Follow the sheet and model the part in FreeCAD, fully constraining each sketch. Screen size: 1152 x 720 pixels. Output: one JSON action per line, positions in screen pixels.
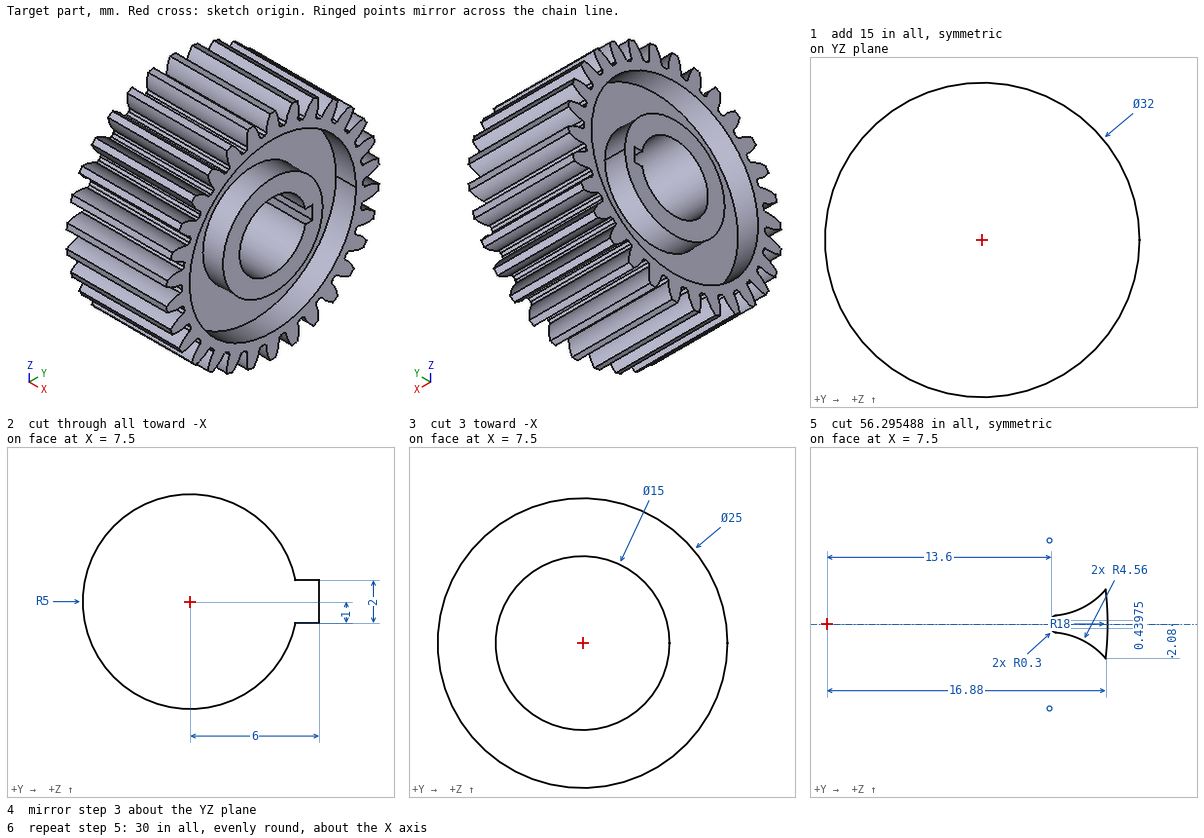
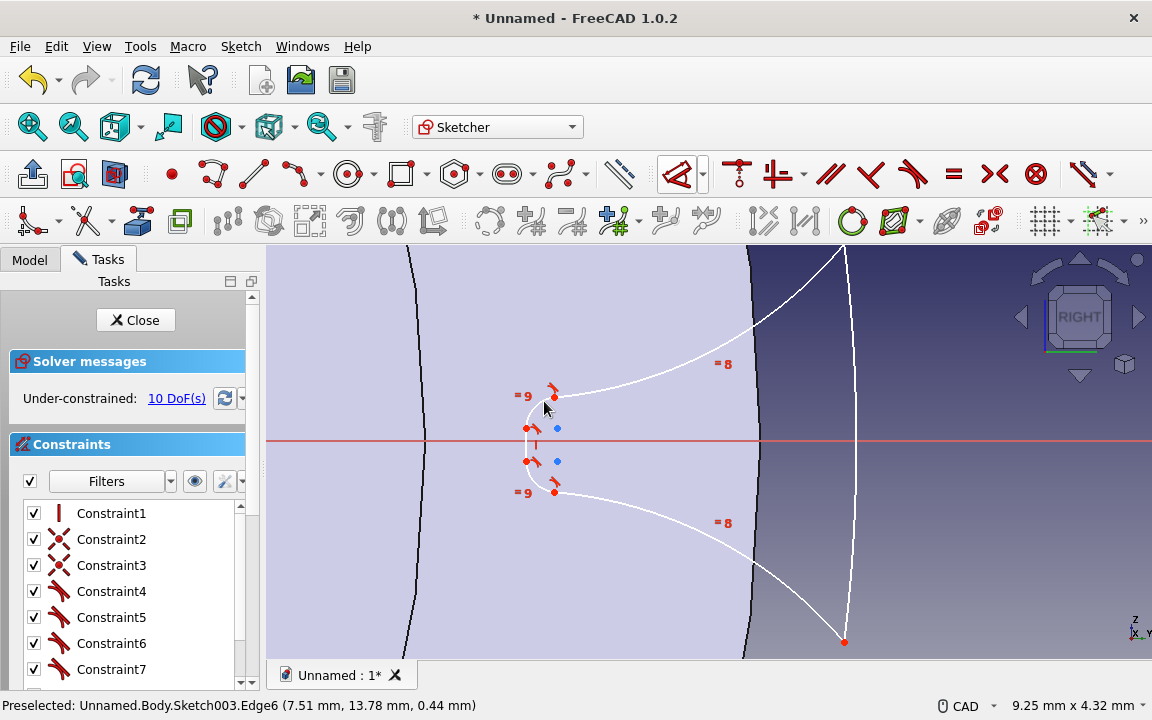
{"action": "scroll", "coordinate": [533, 474], "scroll_direction": "down", "scroll_amount": 2}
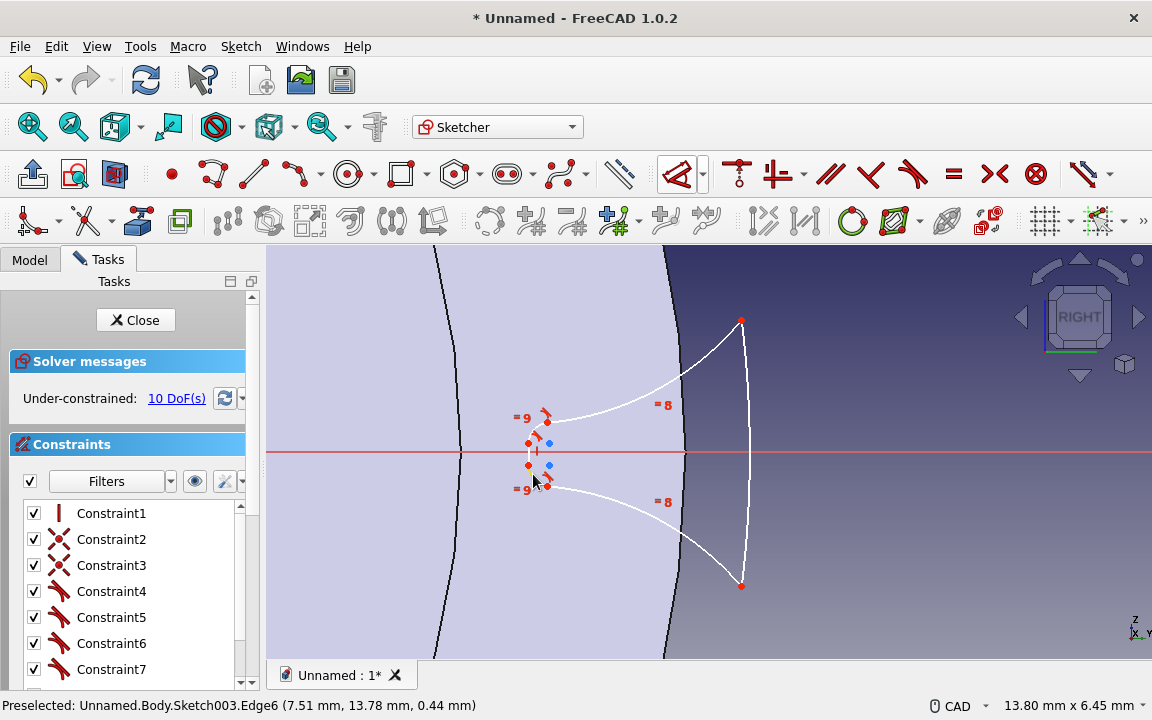
{"action": "scroll", "coordinate": [987, 452], "scroll_direction": "down", "scroll_amount": 4}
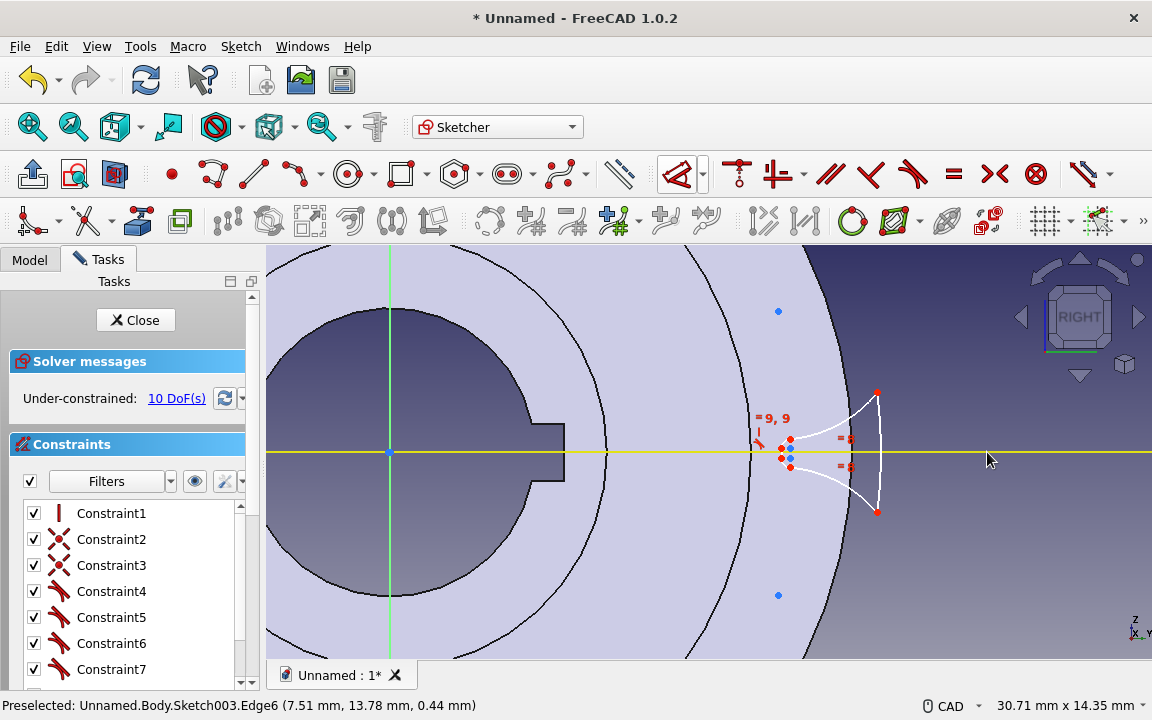
{"action": "scroll", "coordinate": [388, 453], "scroll_direction": "up", "scroll_amount": 9}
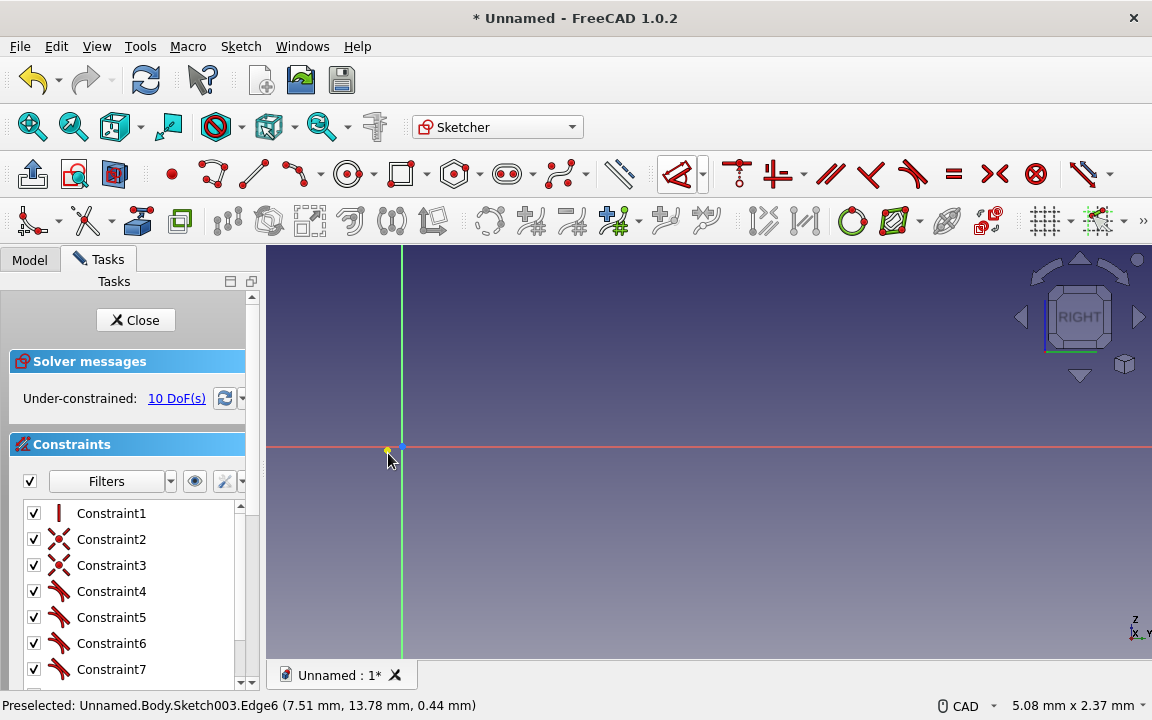
{"action": "left_click", "coordinate": [388, 450]}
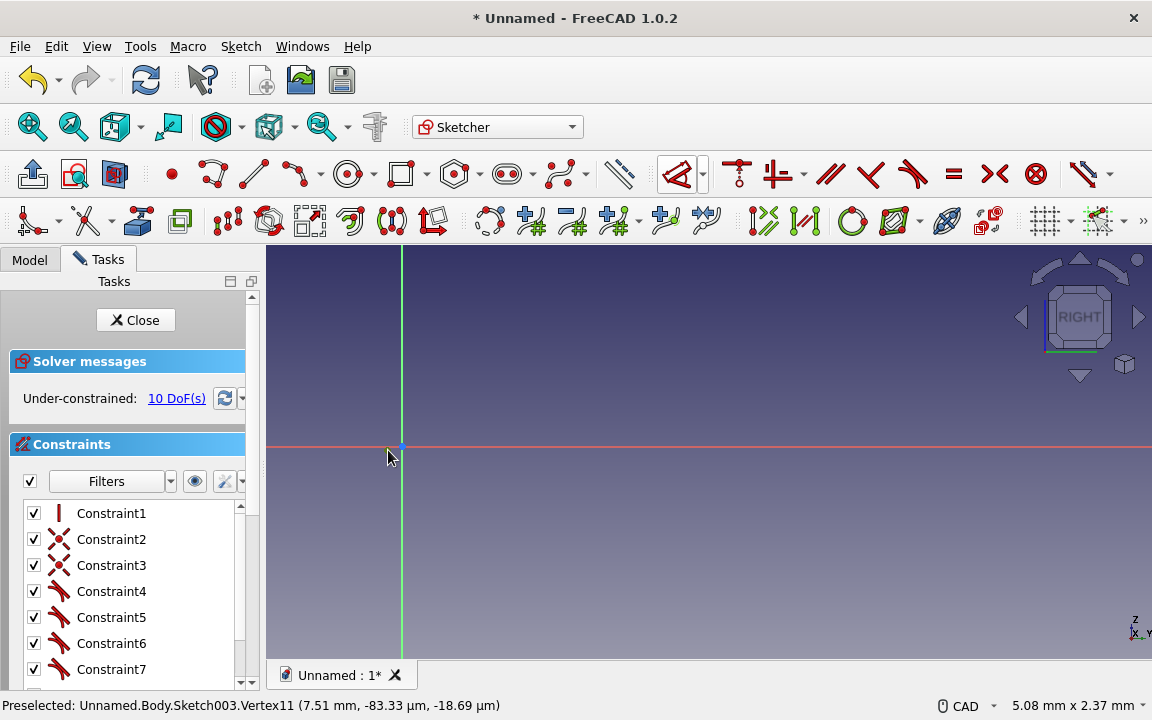
{"action": "left_click", "coordinate": [344, 447]}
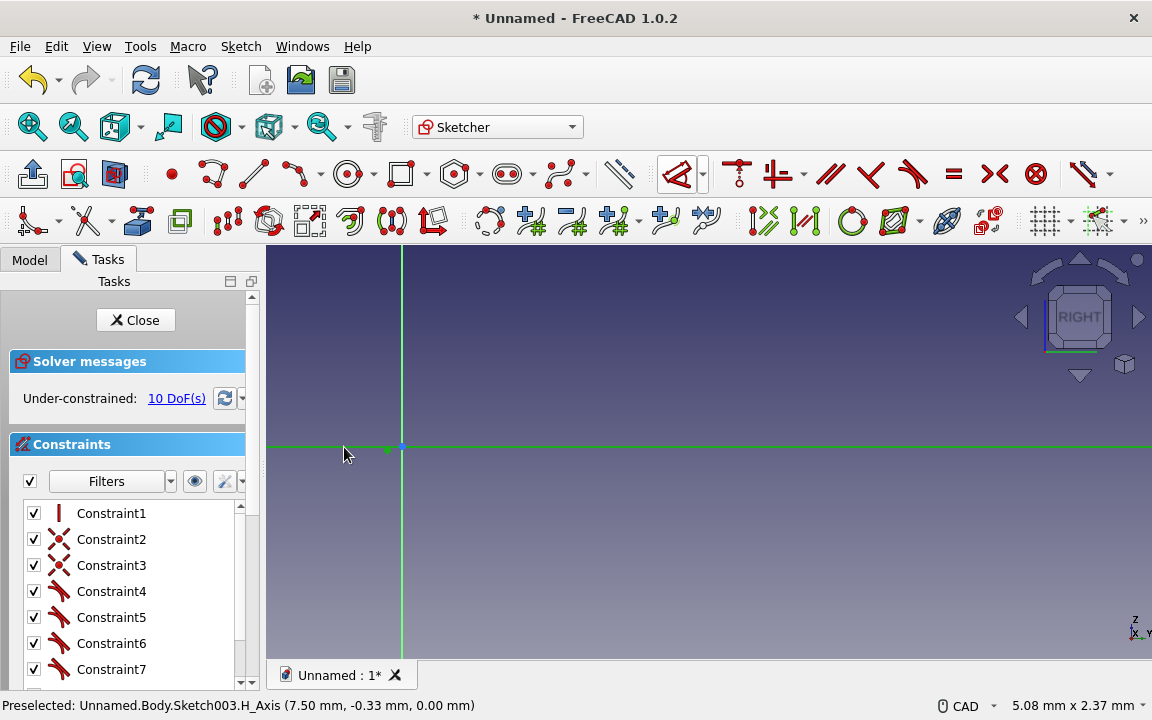
{"action": "key", "text": "c"}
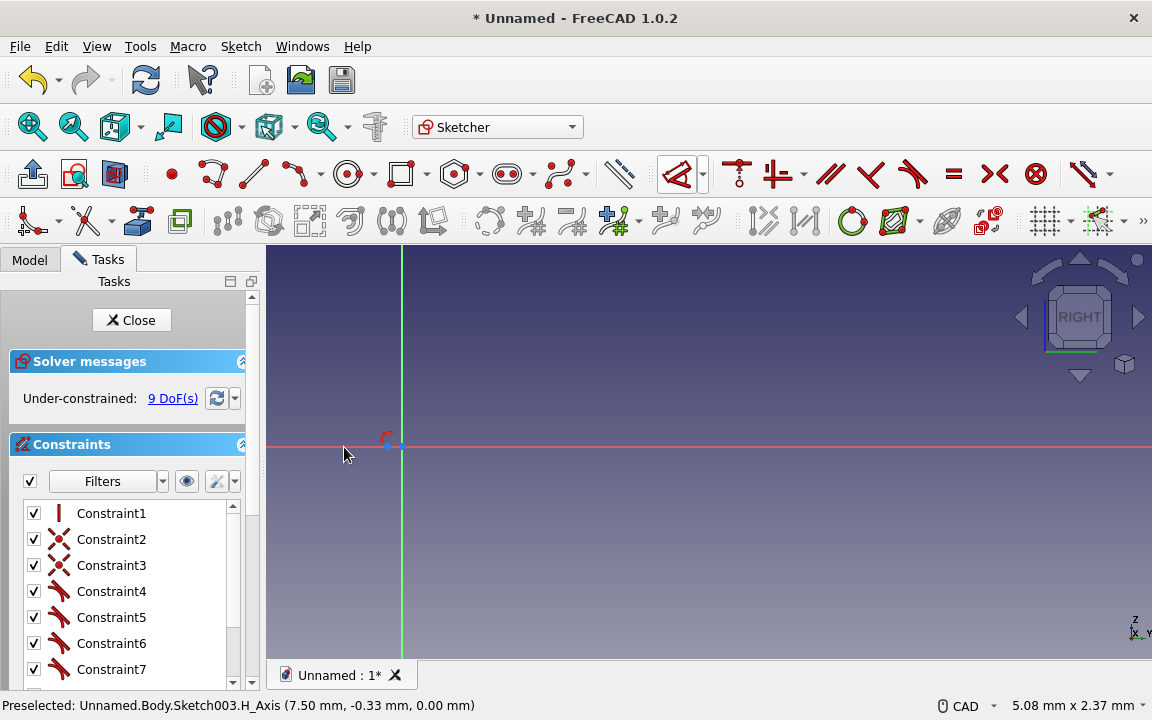
{"action": "scroll", "coordinate": [294, 453], "scroll_direction": "down", "scroll_amount": 8}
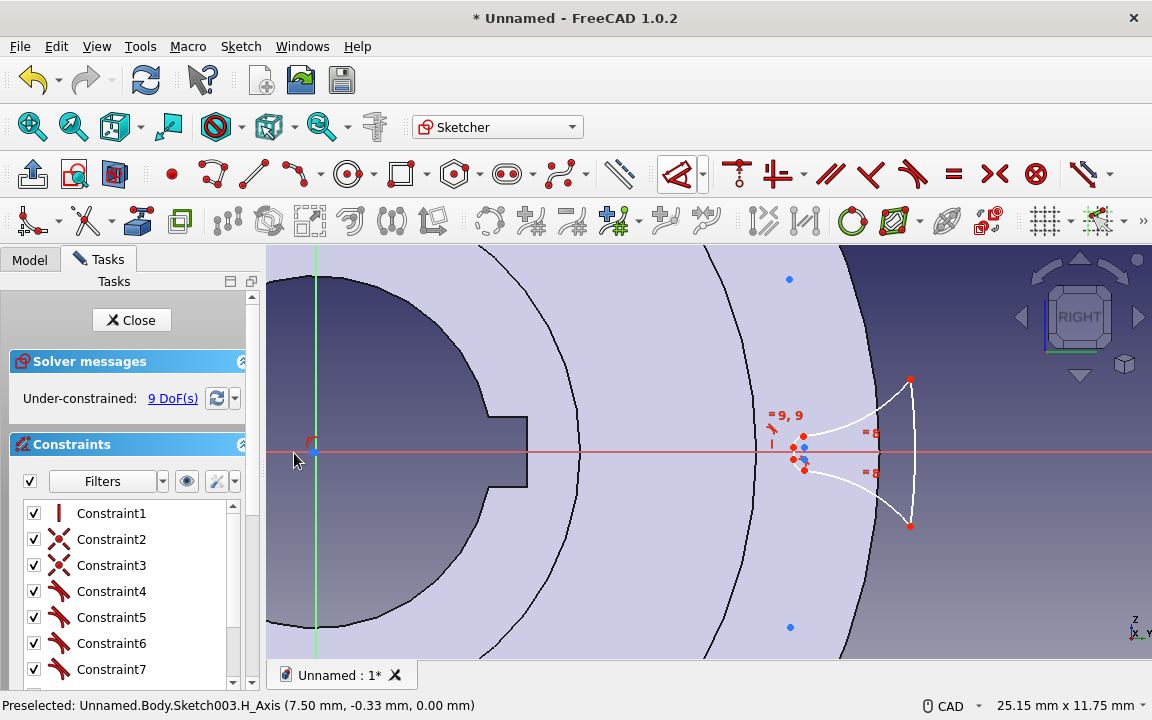
{"action": "scroll", "coordinate": [987, 452], "scroll_direction": "up", "scroll_amount": 3}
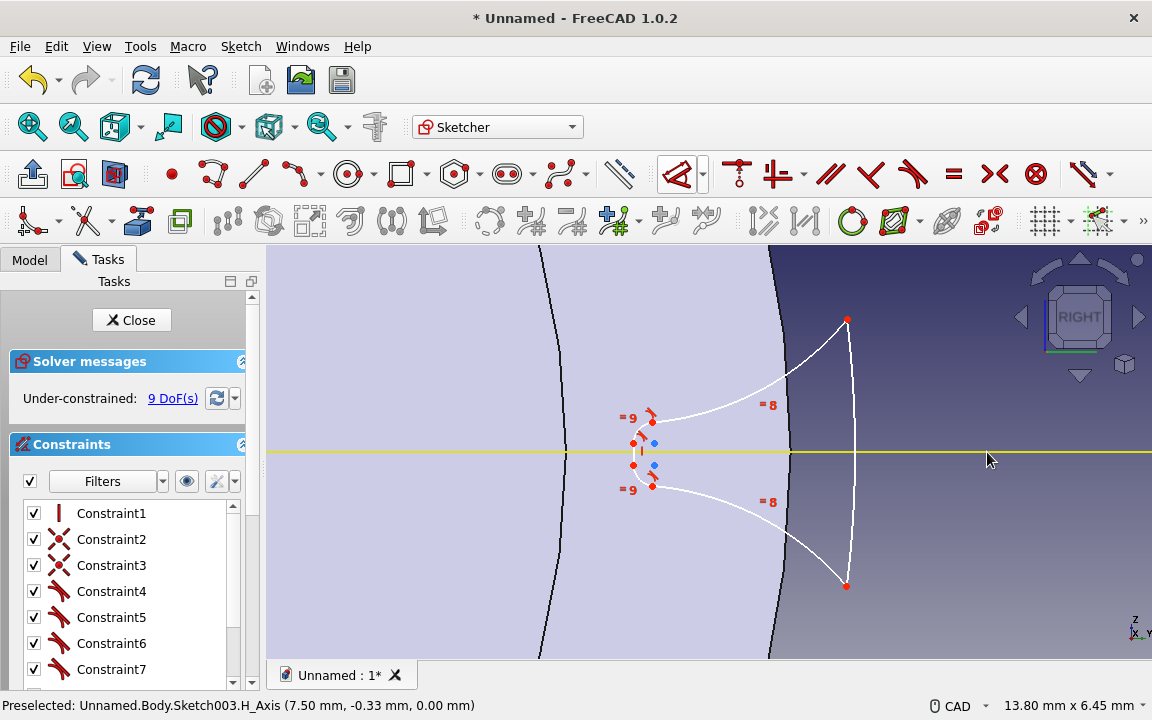
{"action": "scroll", "coordinate": [518, 339], "scroll_direction": "down", "scroll_amount": 3}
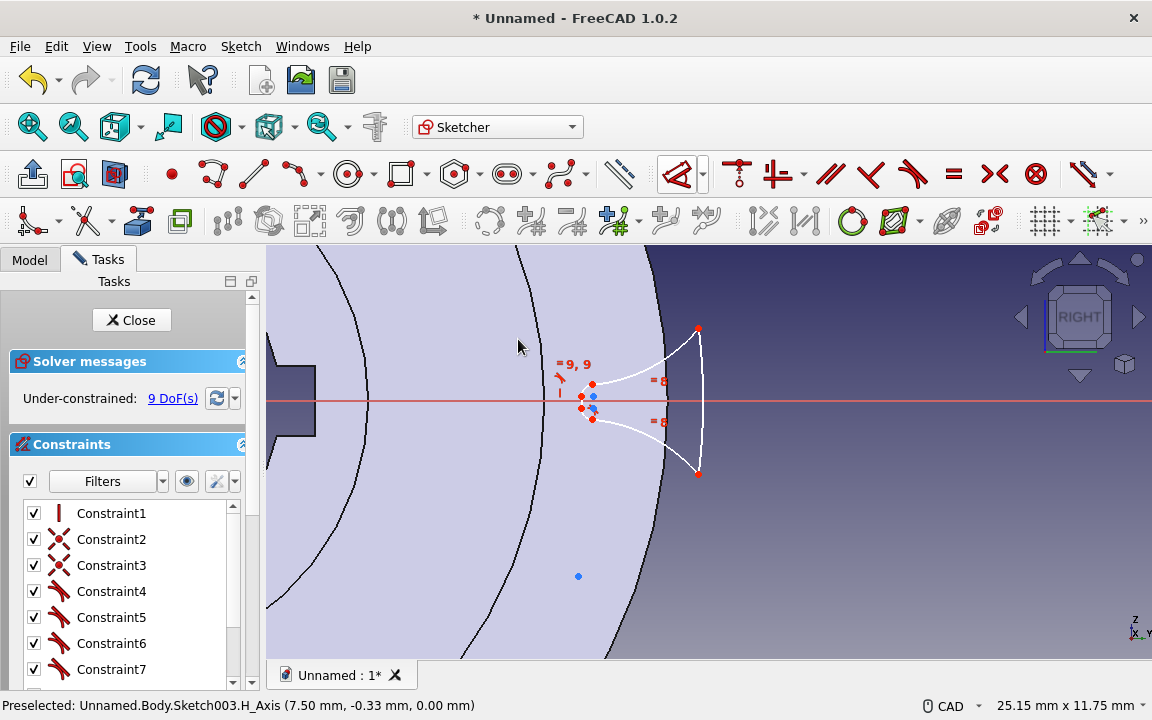
{"action": "left_click", "coordinate": [579, 576]}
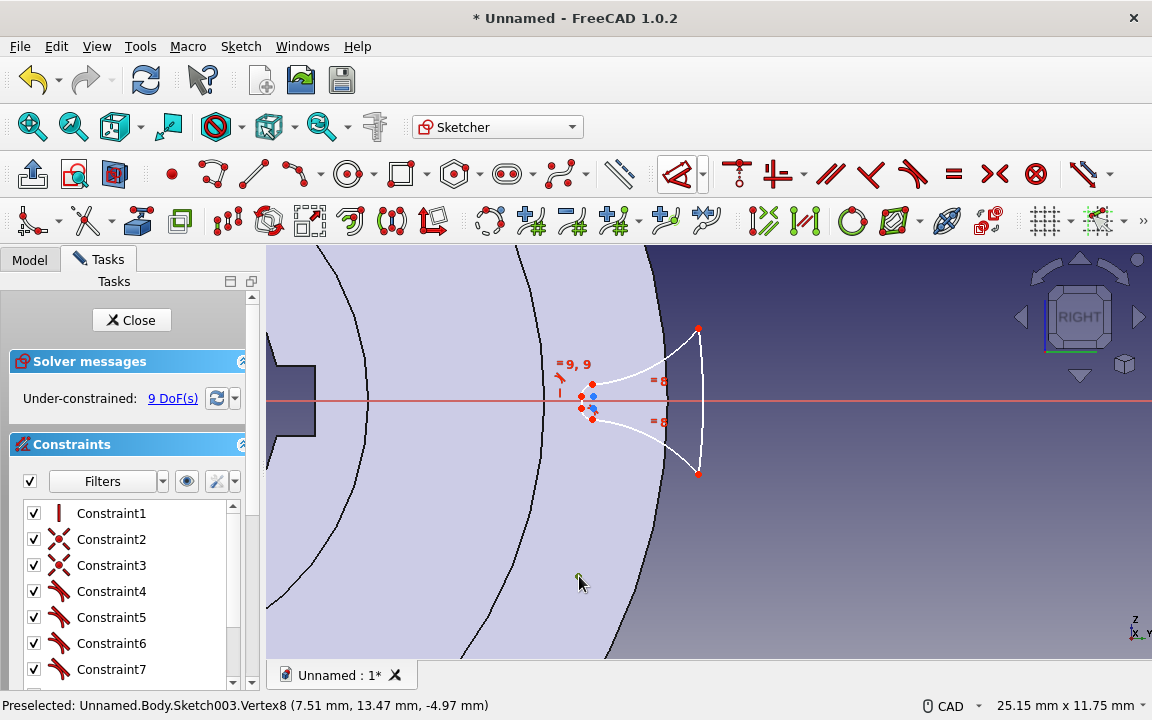
{"action": "scroll", "coordinate": [646, 339], "scroll_direction": "up", "scroll_amount": 3}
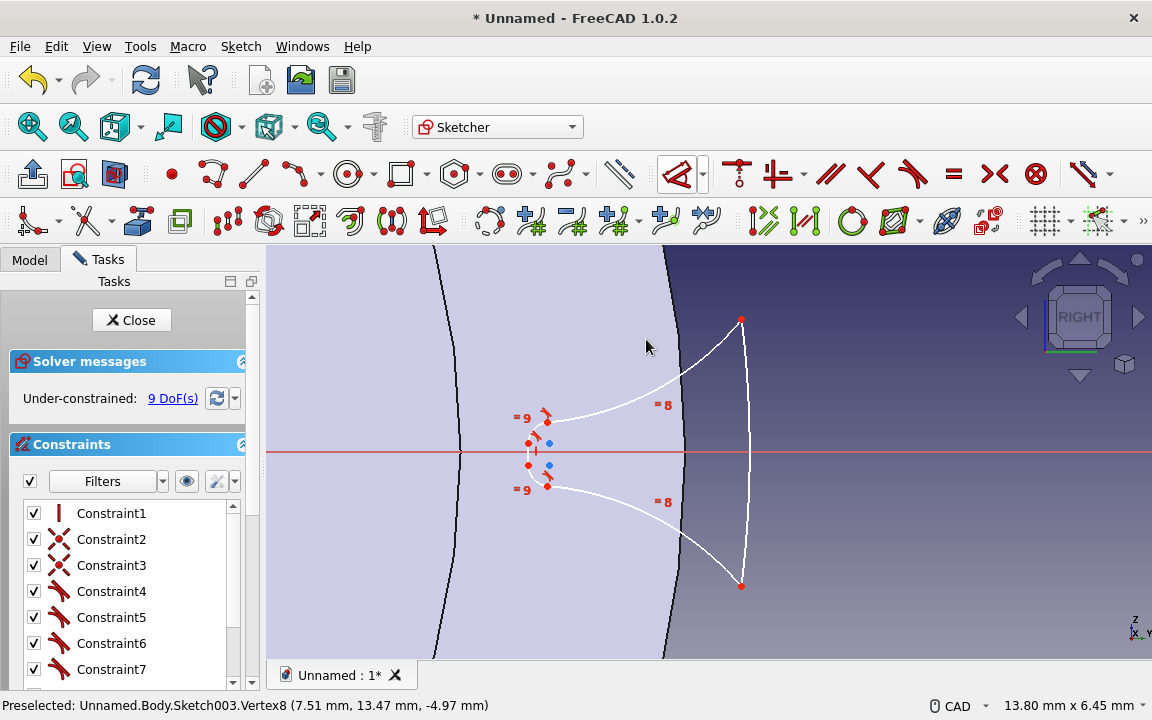
{"action": "scroll", "coordinate": [647, 562], "scroll_direction": "down", "scroll_amount": 3}